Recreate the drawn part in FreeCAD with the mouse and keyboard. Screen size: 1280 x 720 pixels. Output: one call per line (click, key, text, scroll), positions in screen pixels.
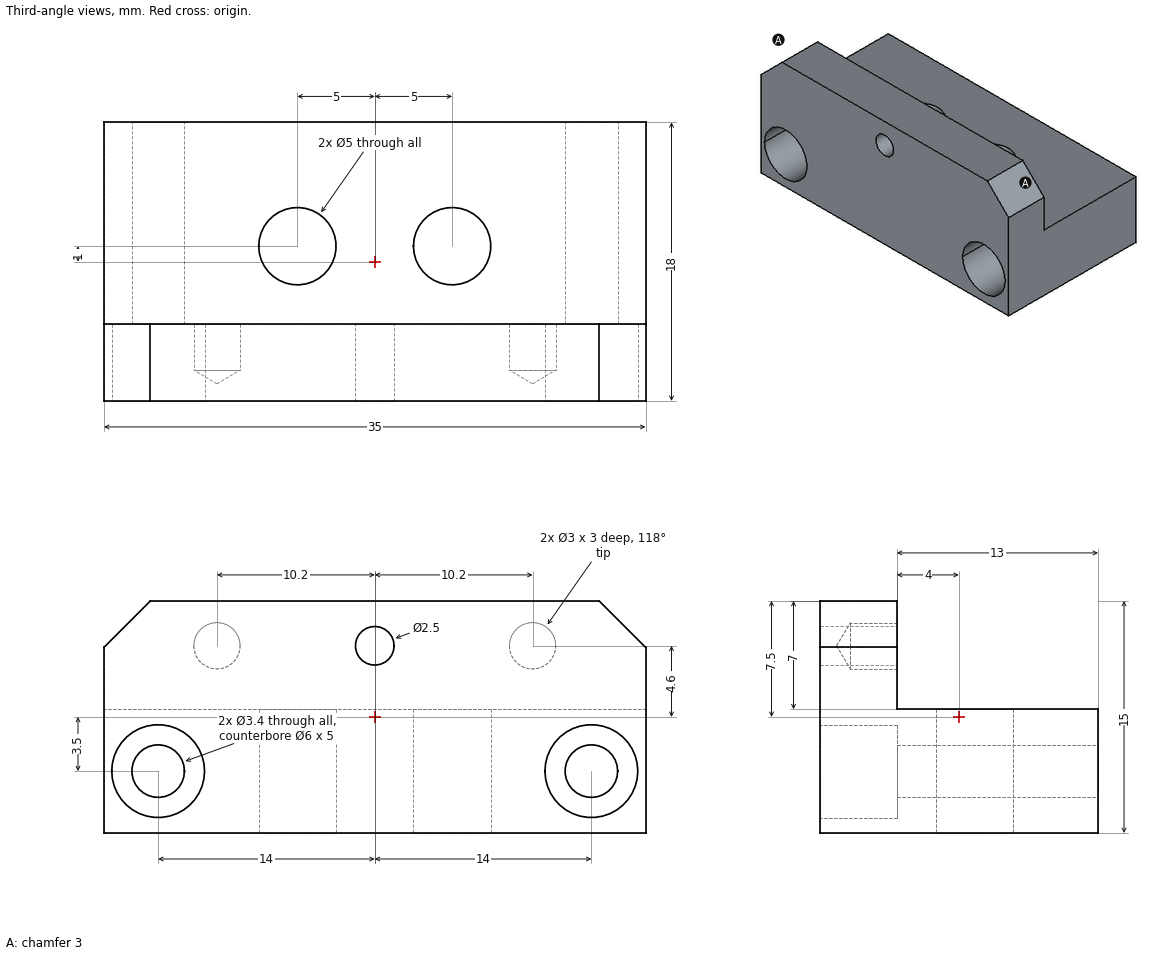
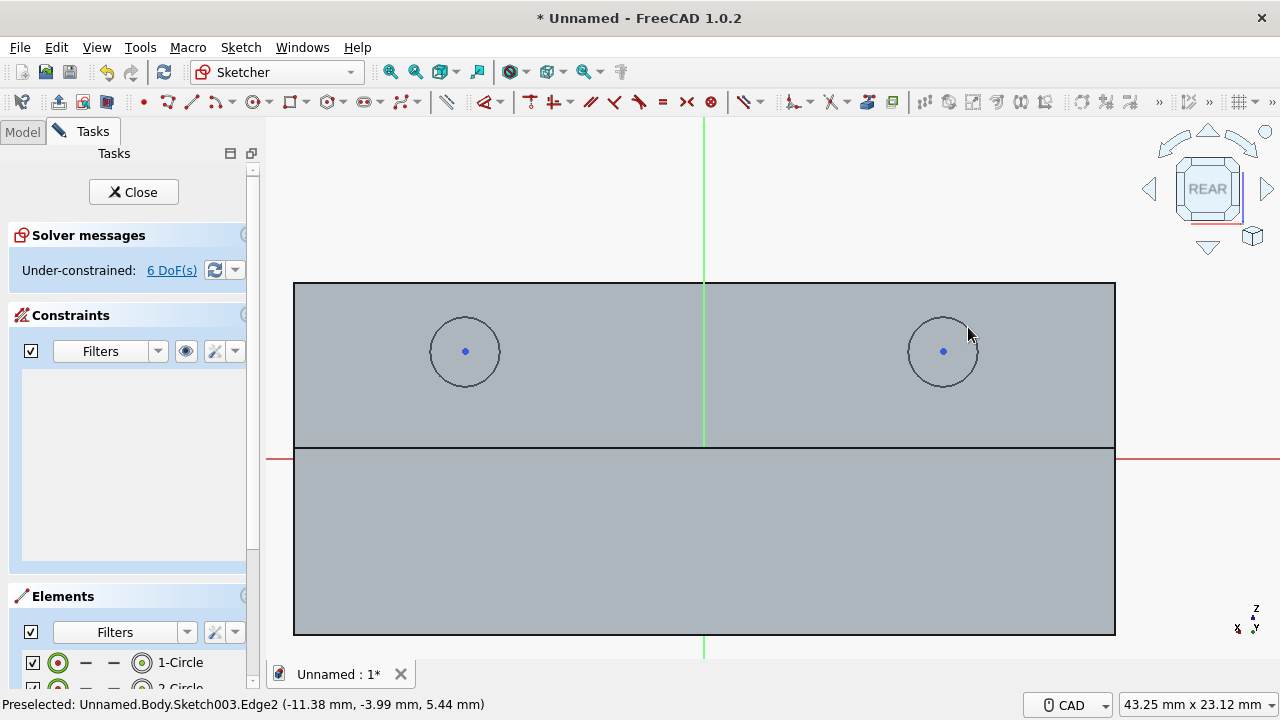
click(489, 327)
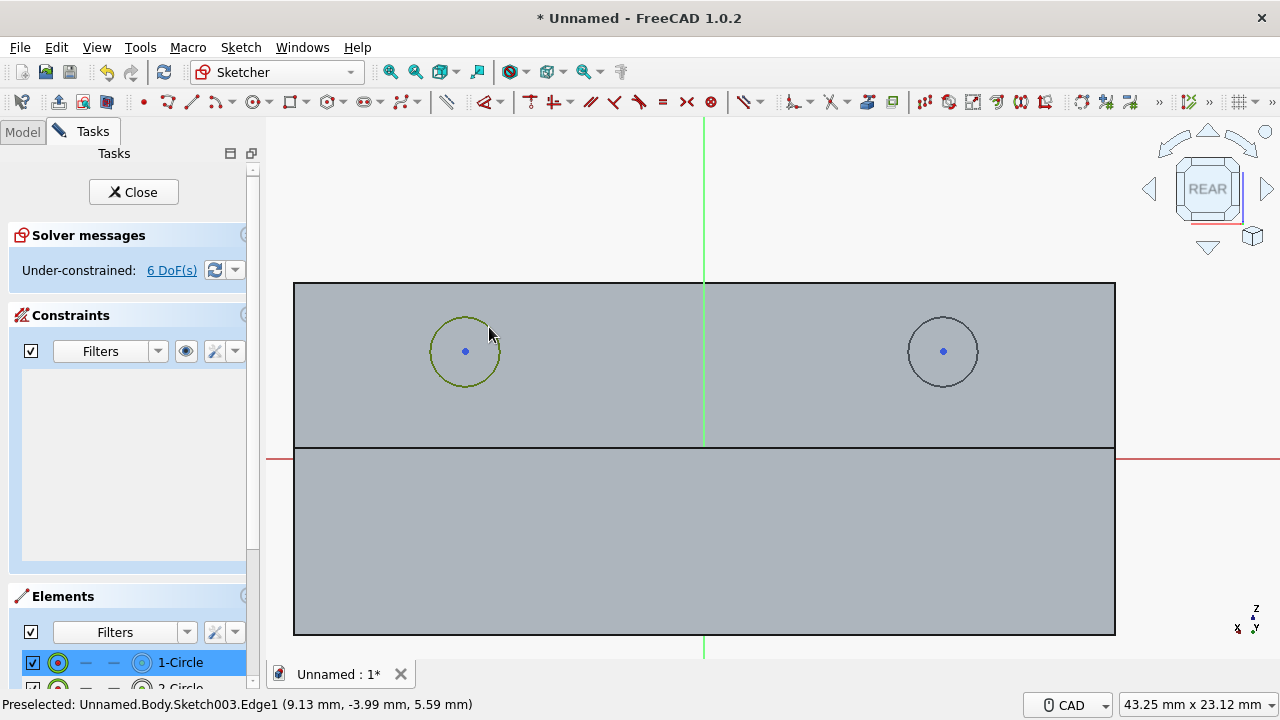
click(967, 327)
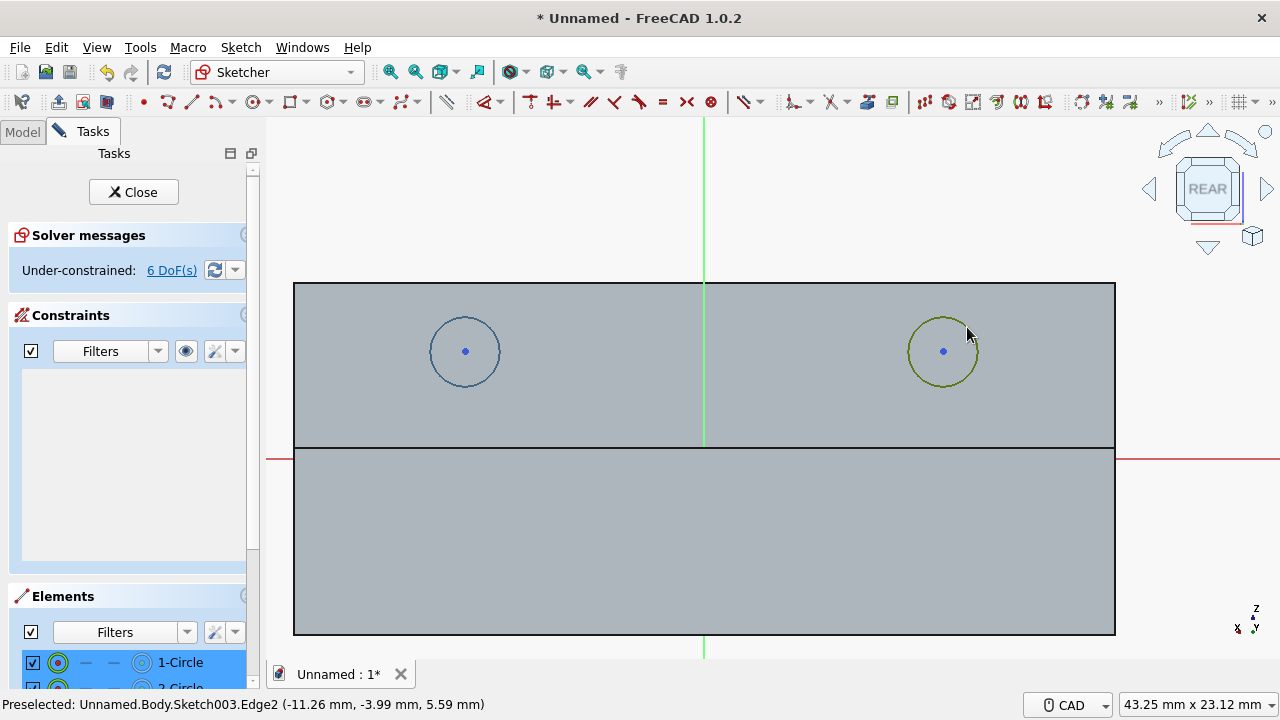
key(e)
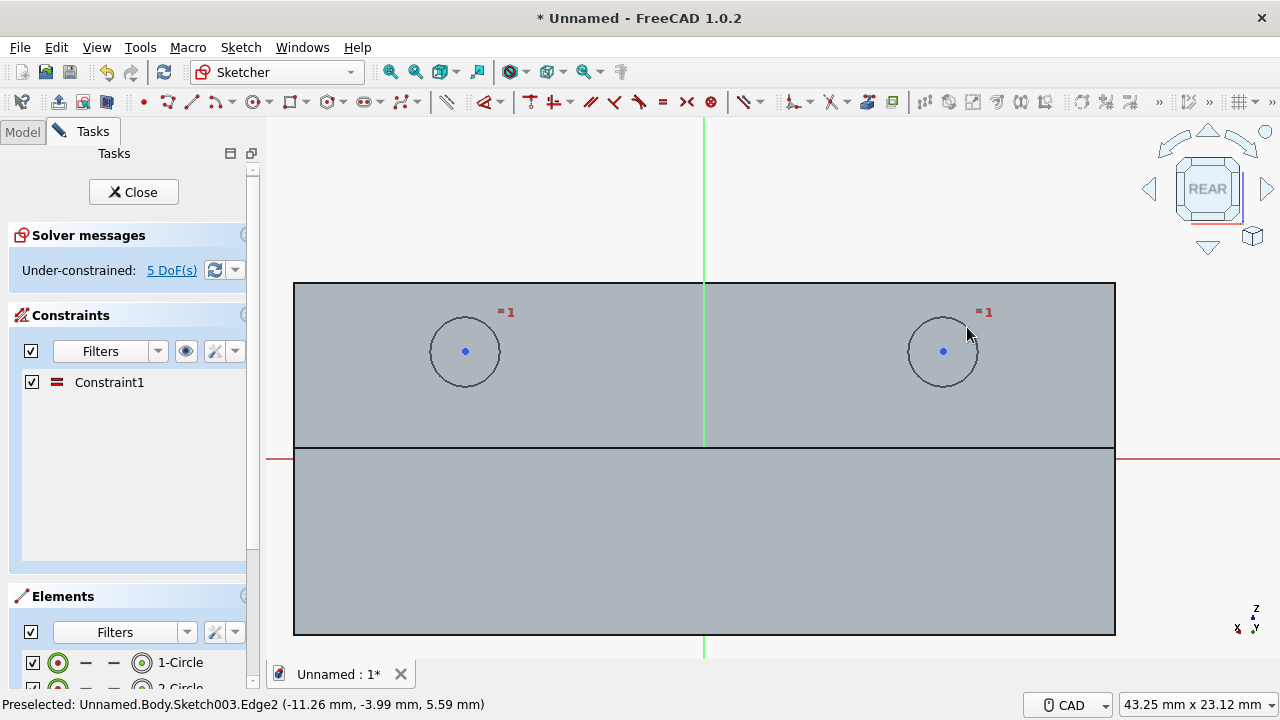
click(465, 352)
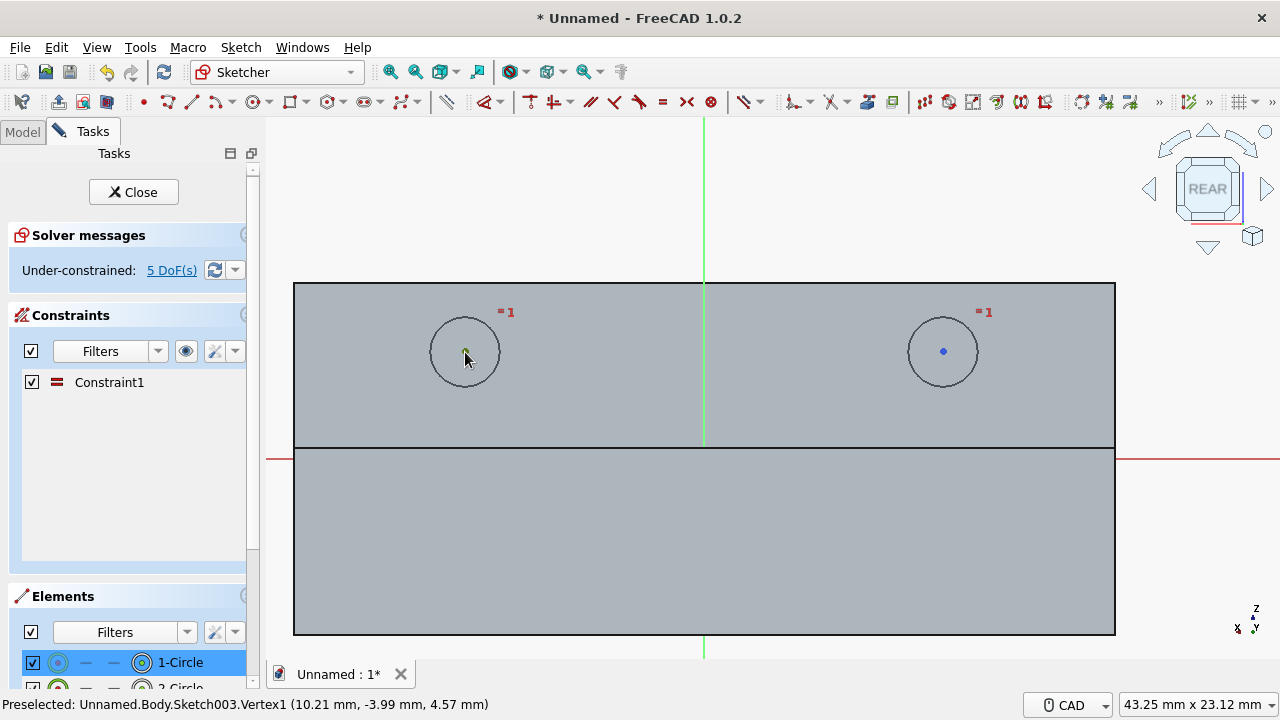
click(943, 352)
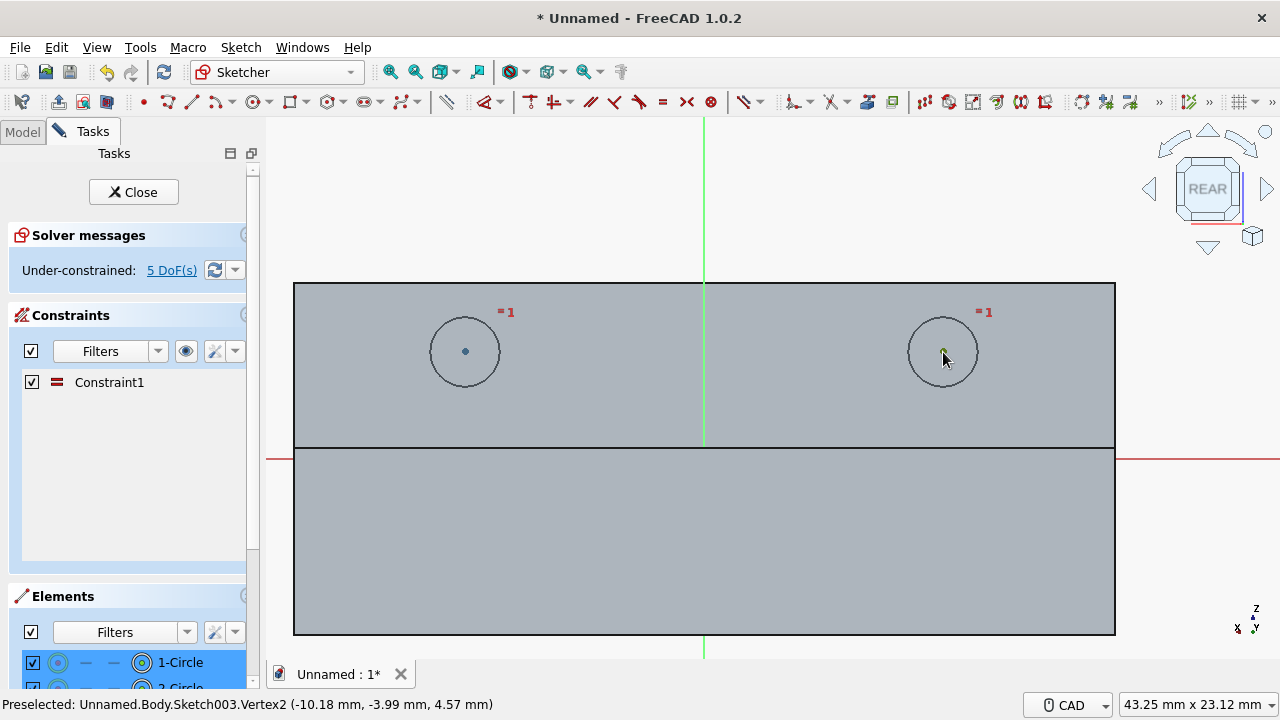
key(h)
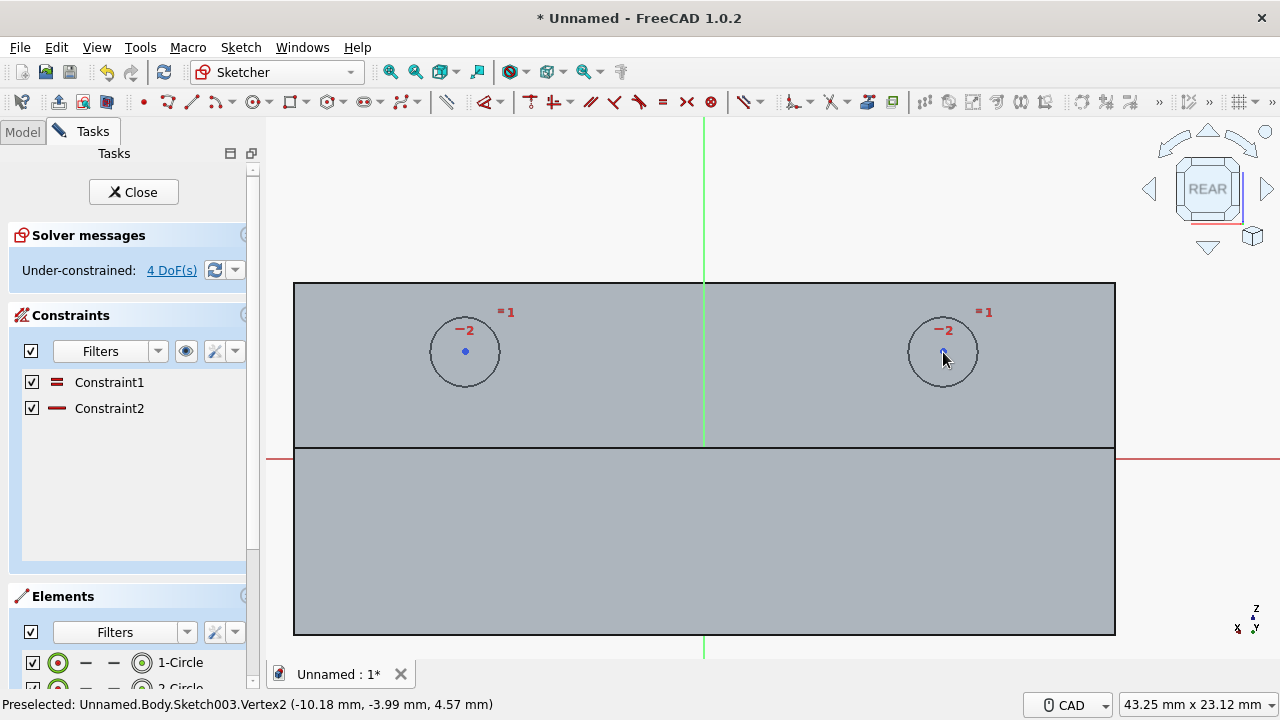
key(d)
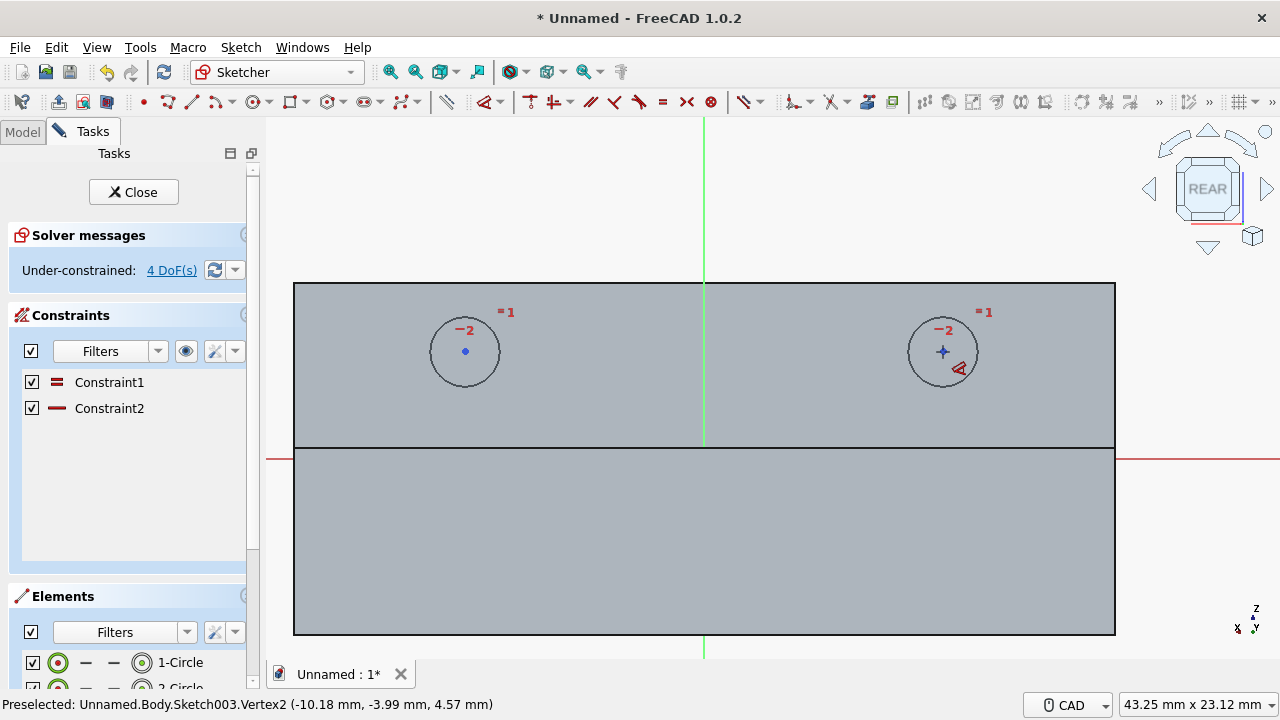
click(489, 327)
click(511, 304)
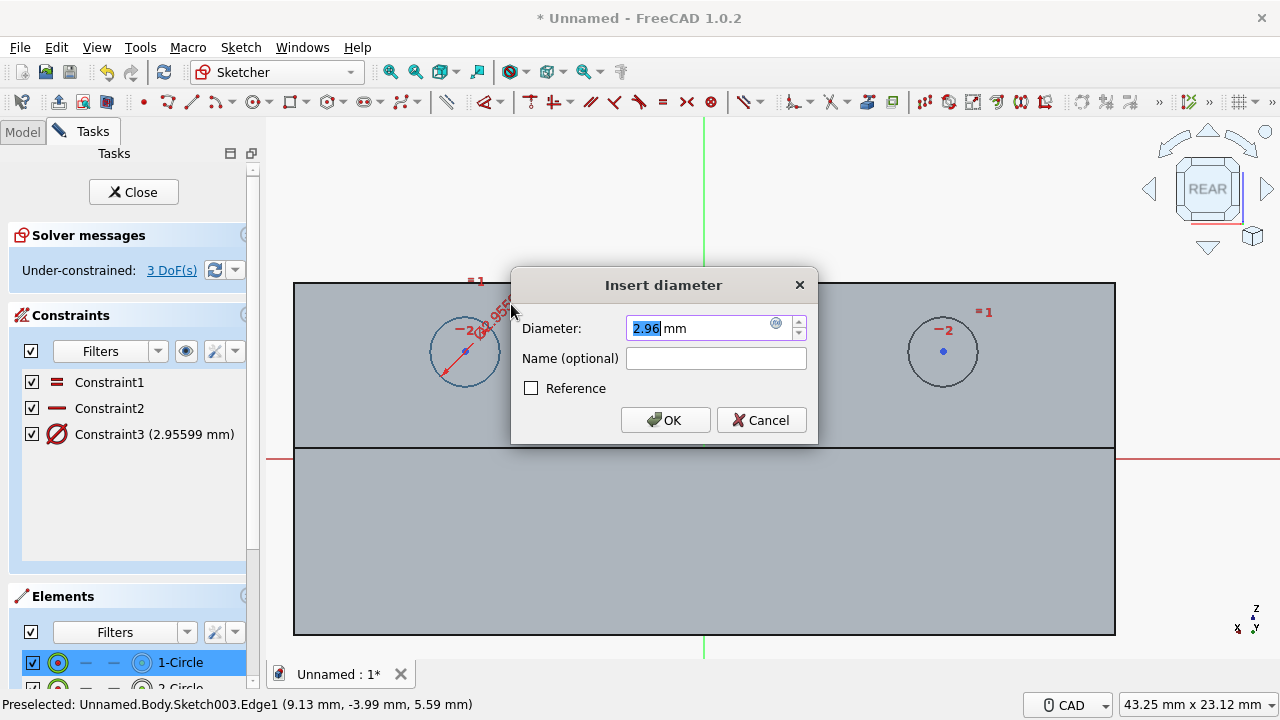
text(3)
key(Return)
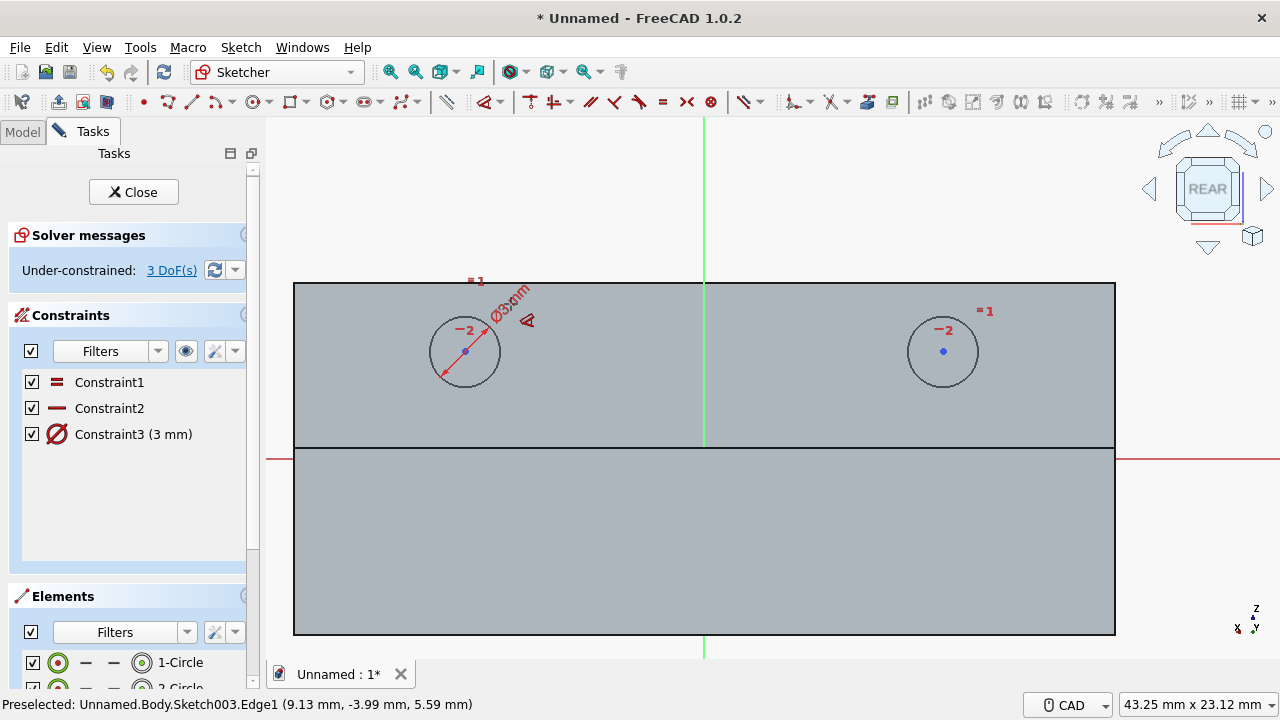
click(465, 352)
click(431, 406)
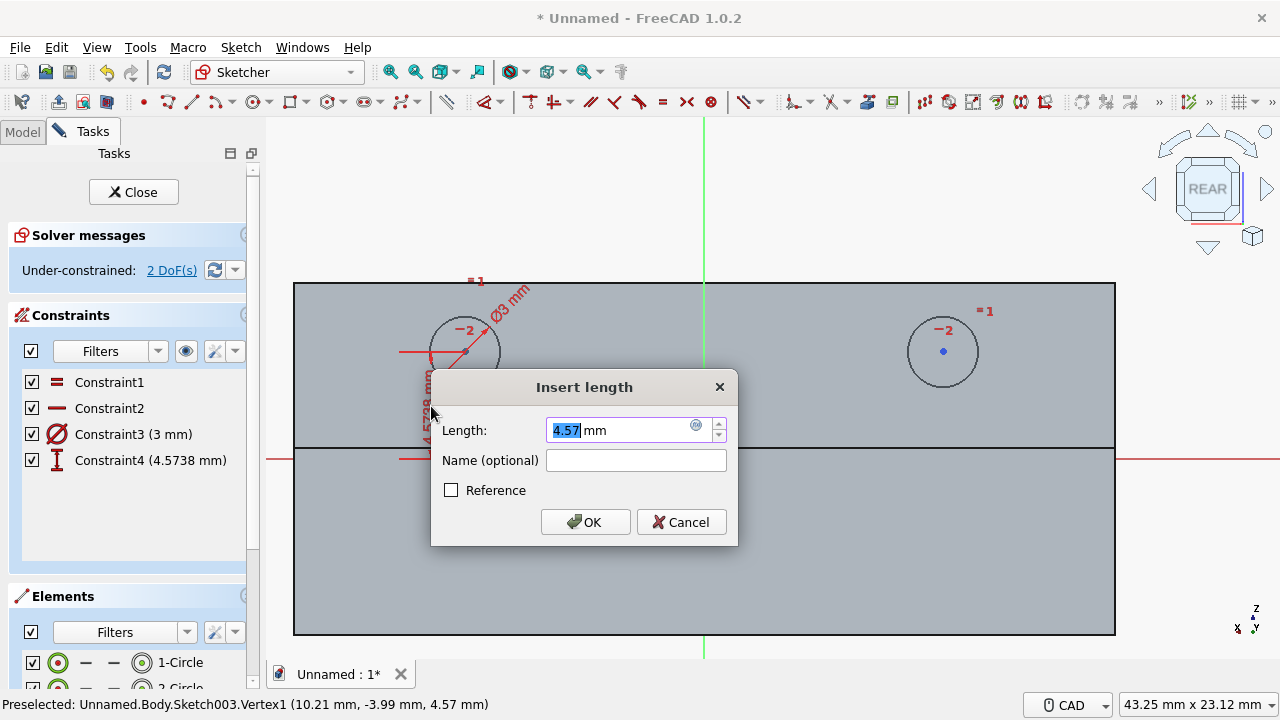
text(4.6)
key(Return)